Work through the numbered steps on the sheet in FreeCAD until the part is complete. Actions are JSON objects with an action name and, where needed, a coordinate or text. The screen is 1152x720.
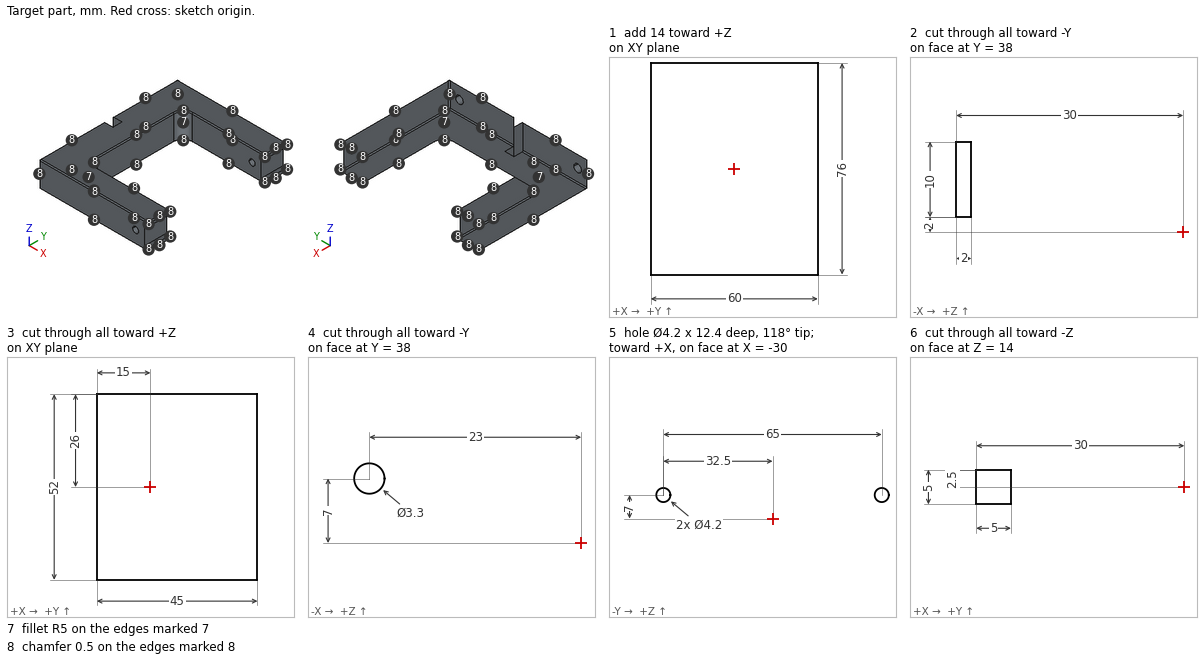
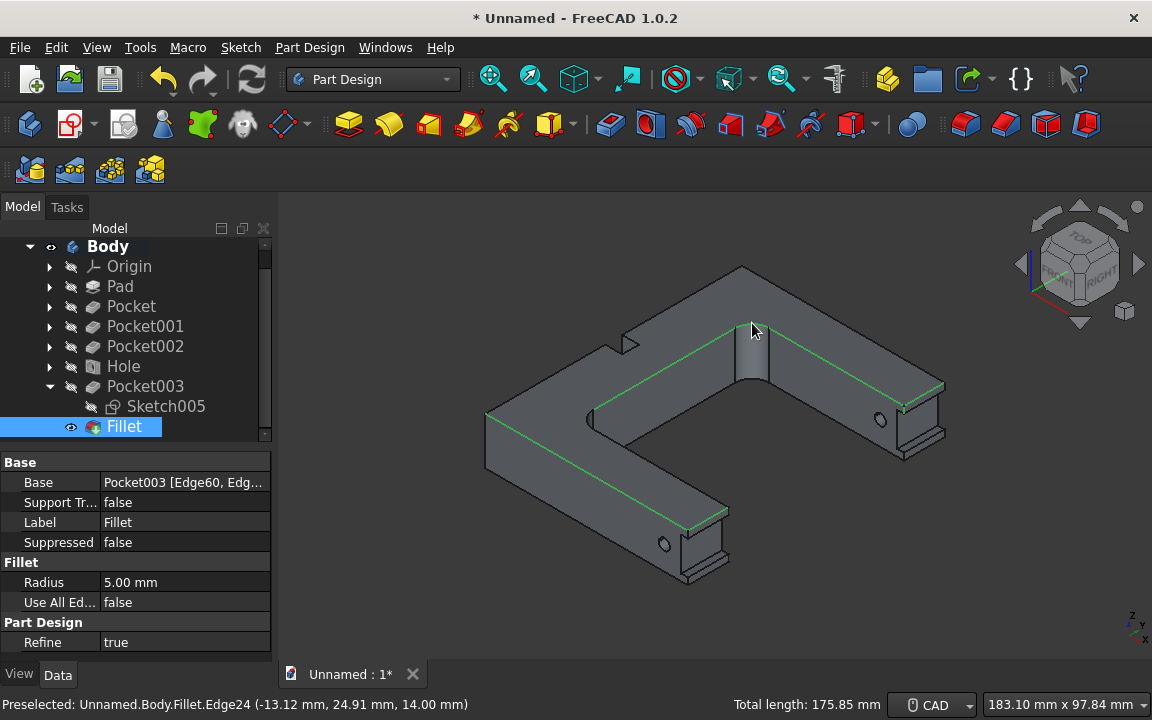
{"action": "left_click", "coordinate": [587, 419], "text": "ctrl"}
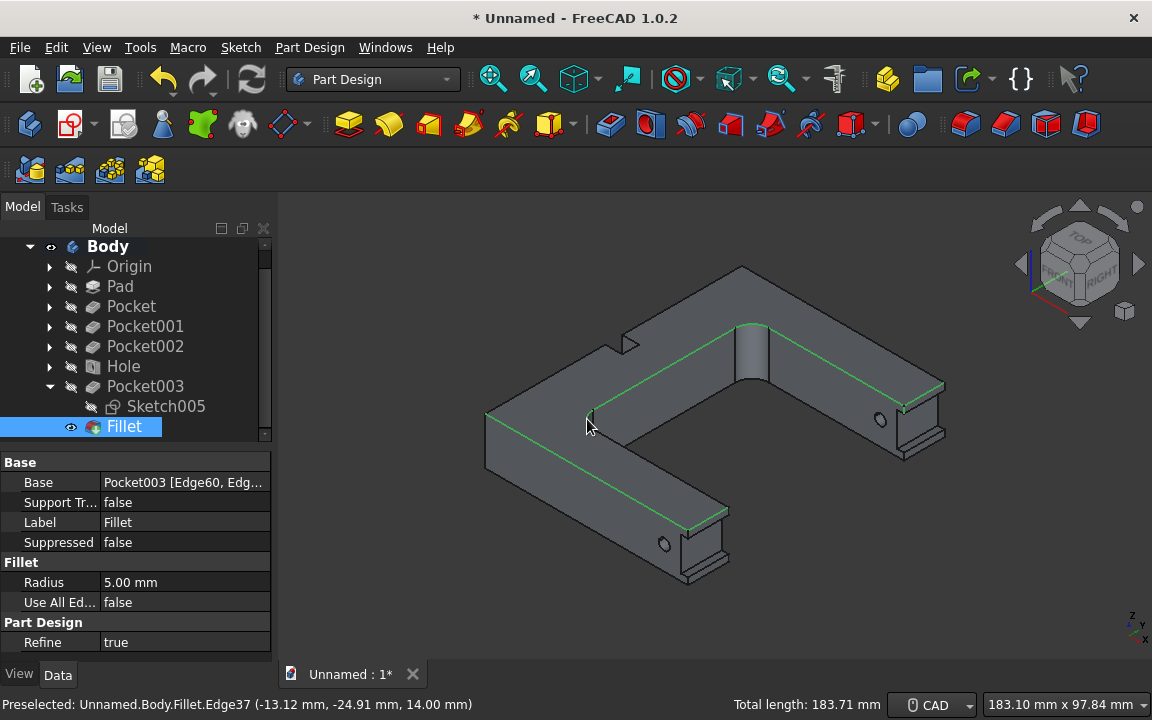
{"action": "key", "text": "2"}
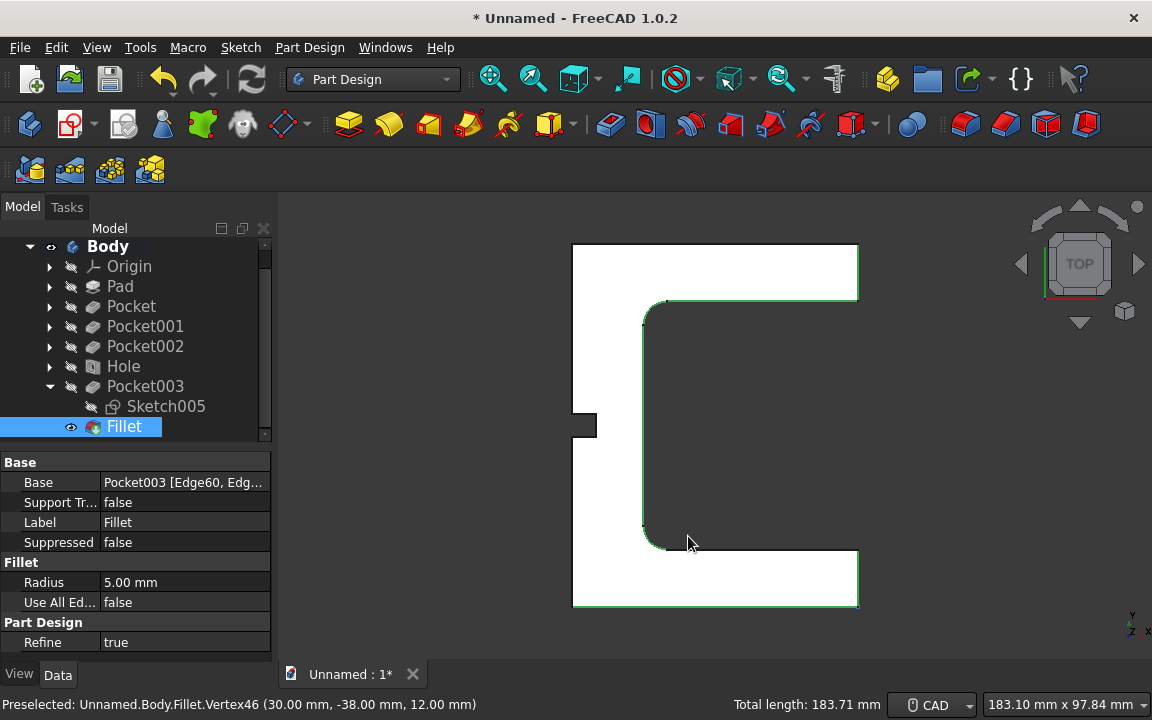
{"action": "left_click", "coordinate": [572, 328], "text": "ctrl"}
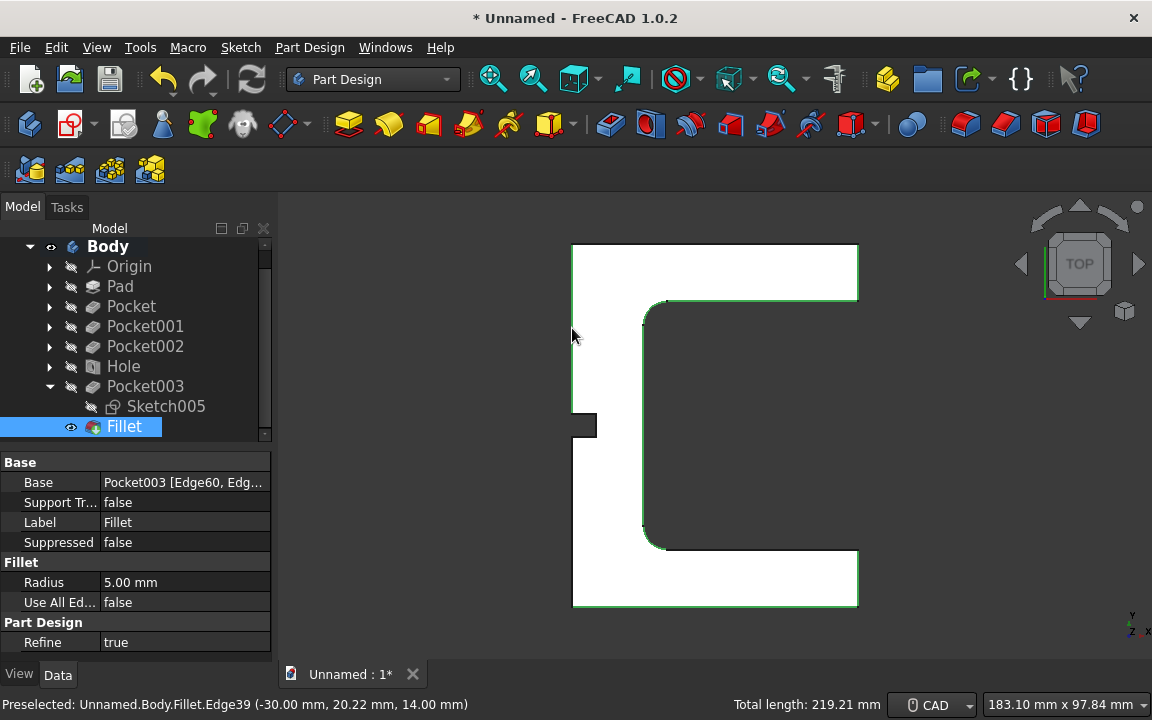
{"action": "left_click", "coordinate": [763, 549], "text": "ctrl"}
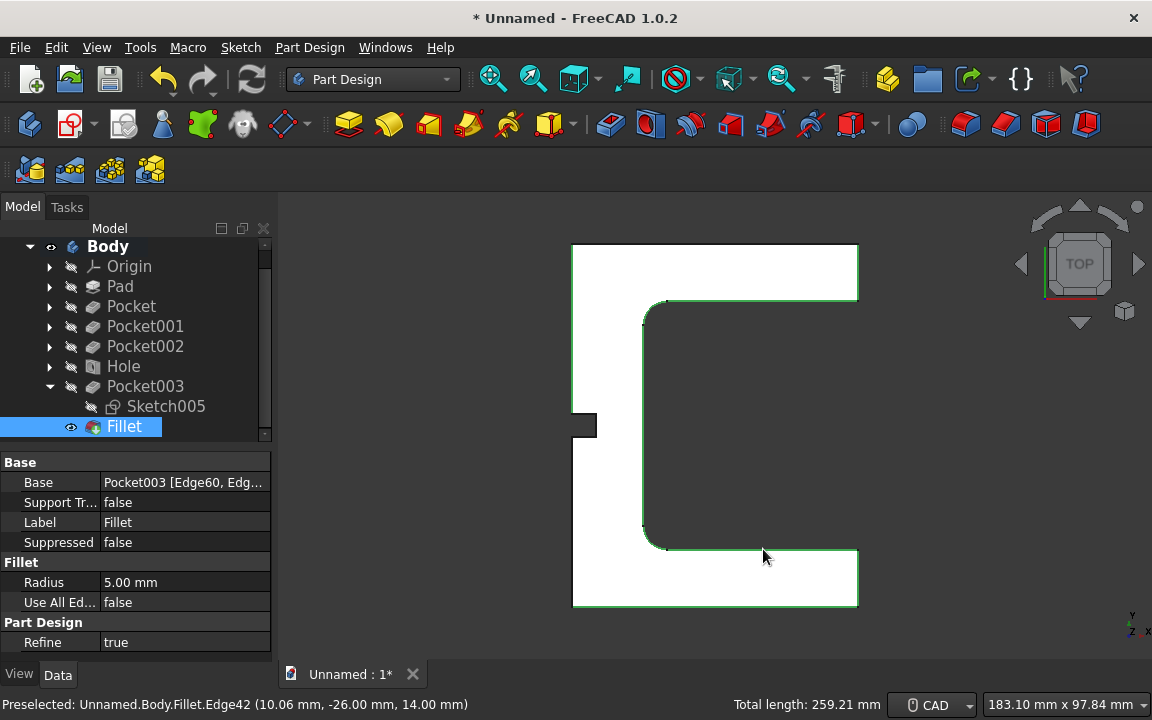
{"action": "left_click", "coordinate": [572, 521], "text": "ctrl"}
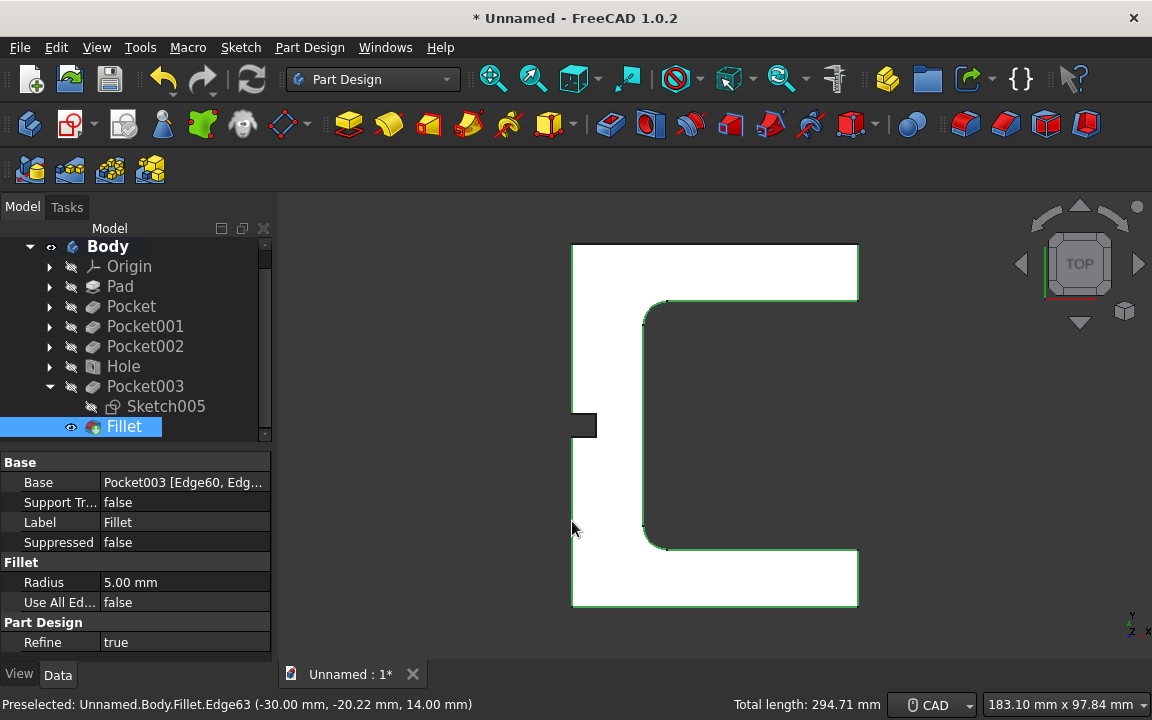
{"action": "left_click", "coordinate": [715, 243], "text": "ctrl"}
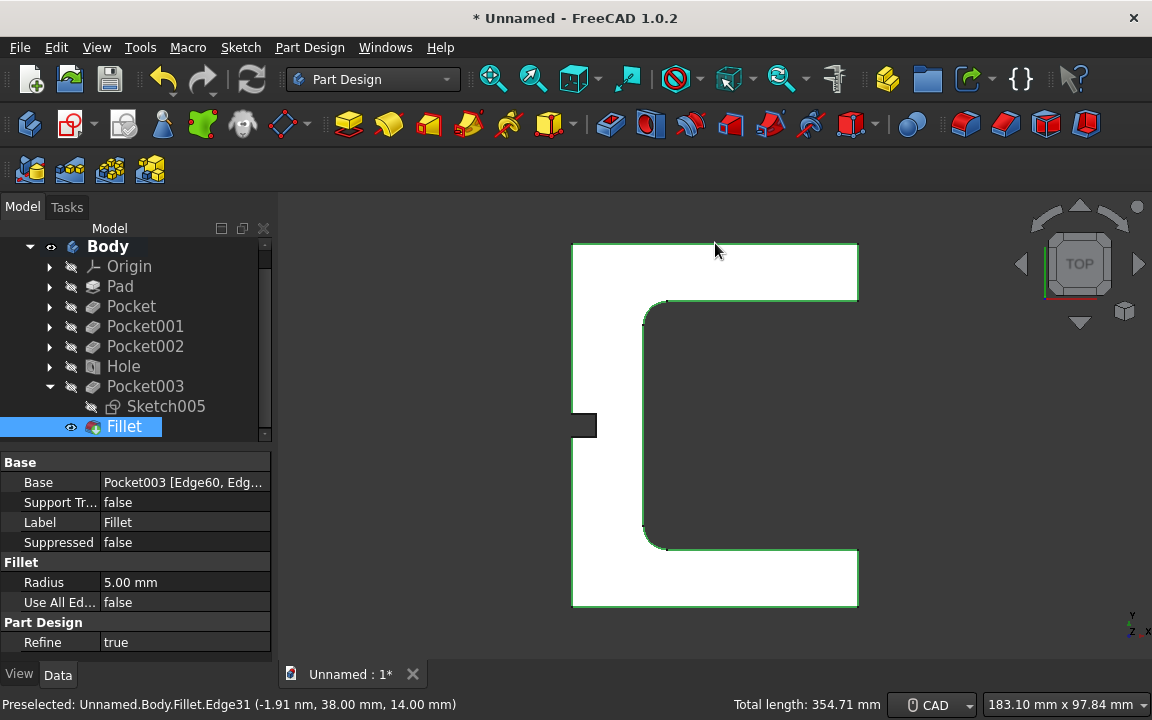
{"action": "scroll", "coordinate": [858, 606], "scroll_direction": "up", "scroll_amount": 8}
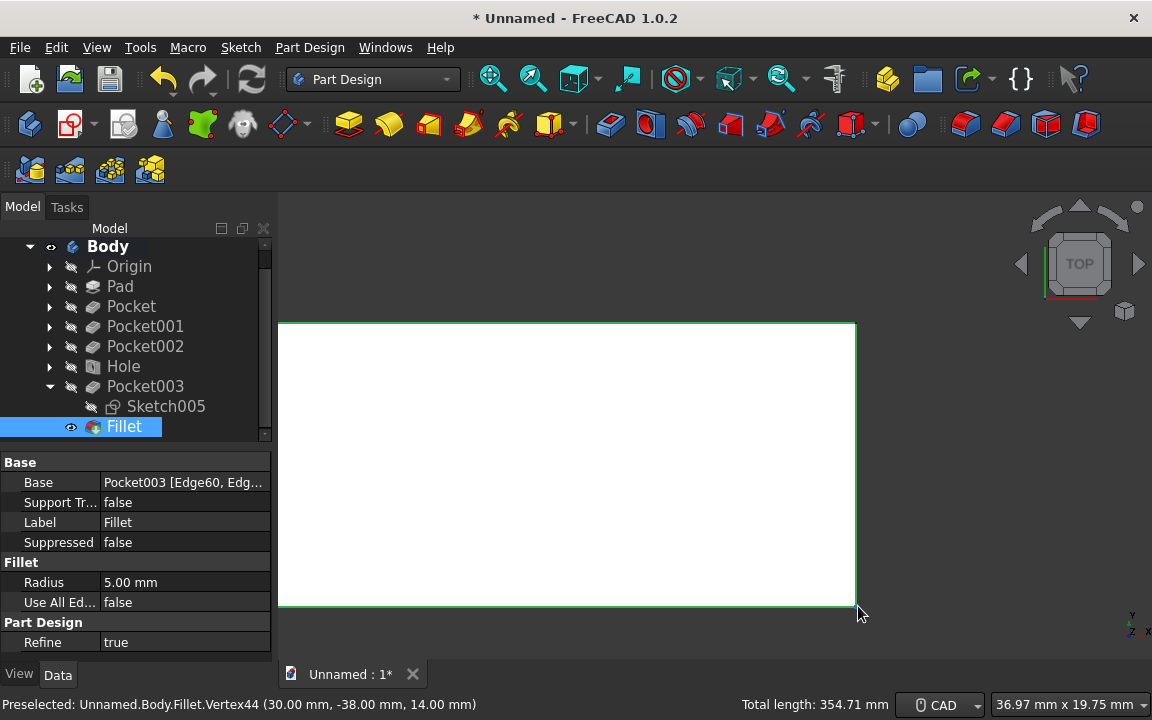
{"action": "left_click", "coordinate": [494, 80]}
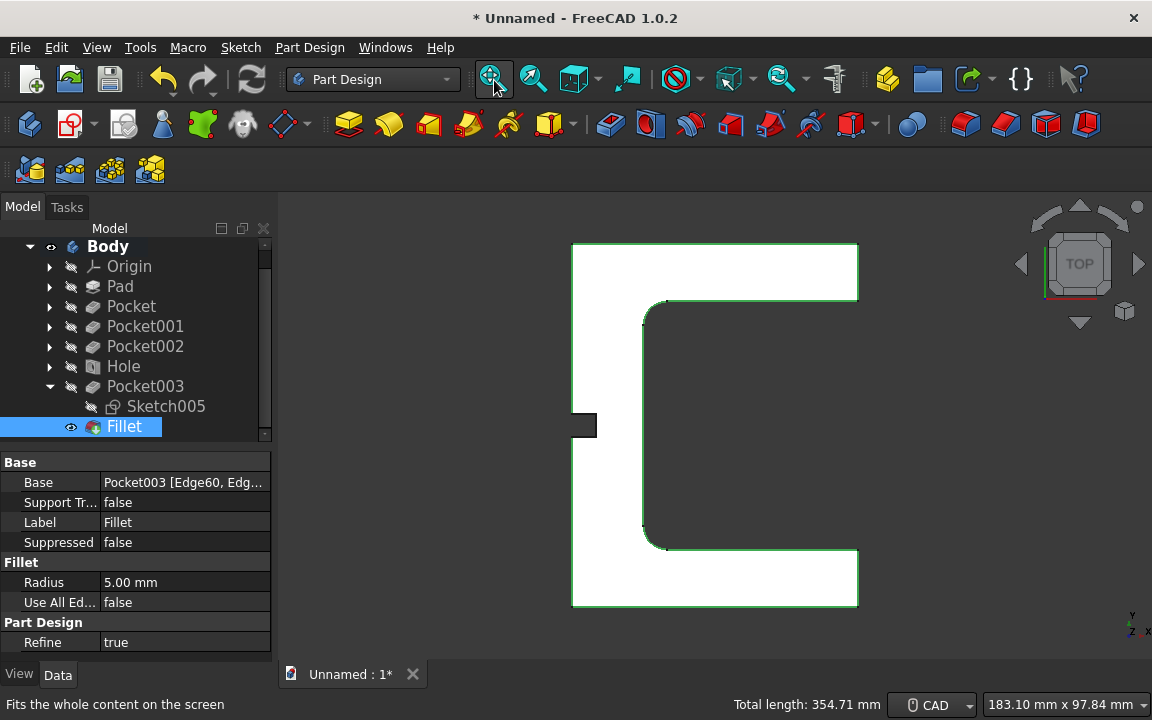
{"action": "key", "text": "0"}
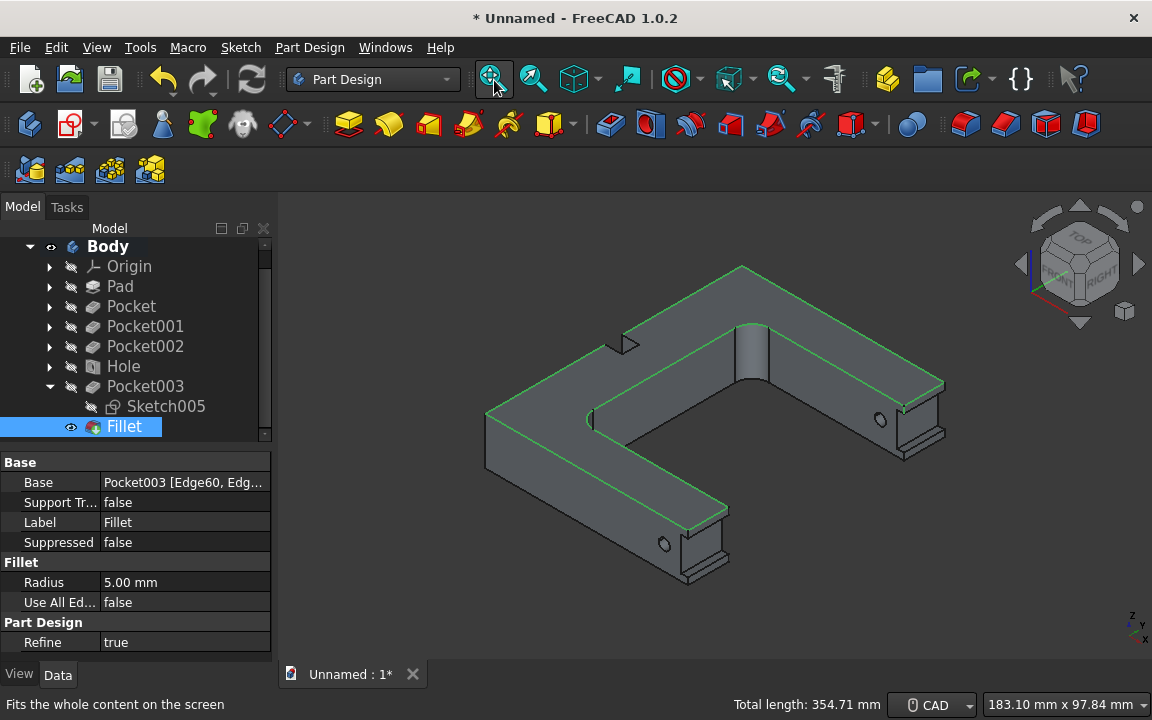
{"action": "scroll", "coordinate": [688, 580], "scroll_direction": "up", "scroll_amount": 8}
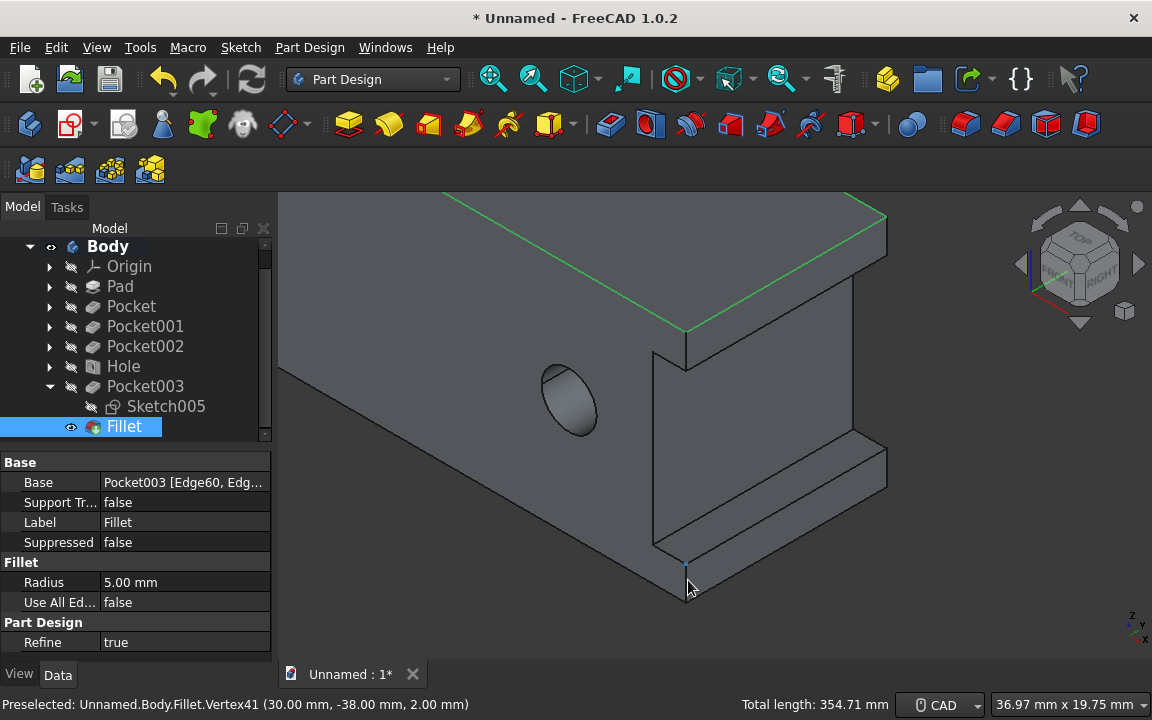
{"action": "left_click", "coordinate": [686, 583], "text": "ctrl"}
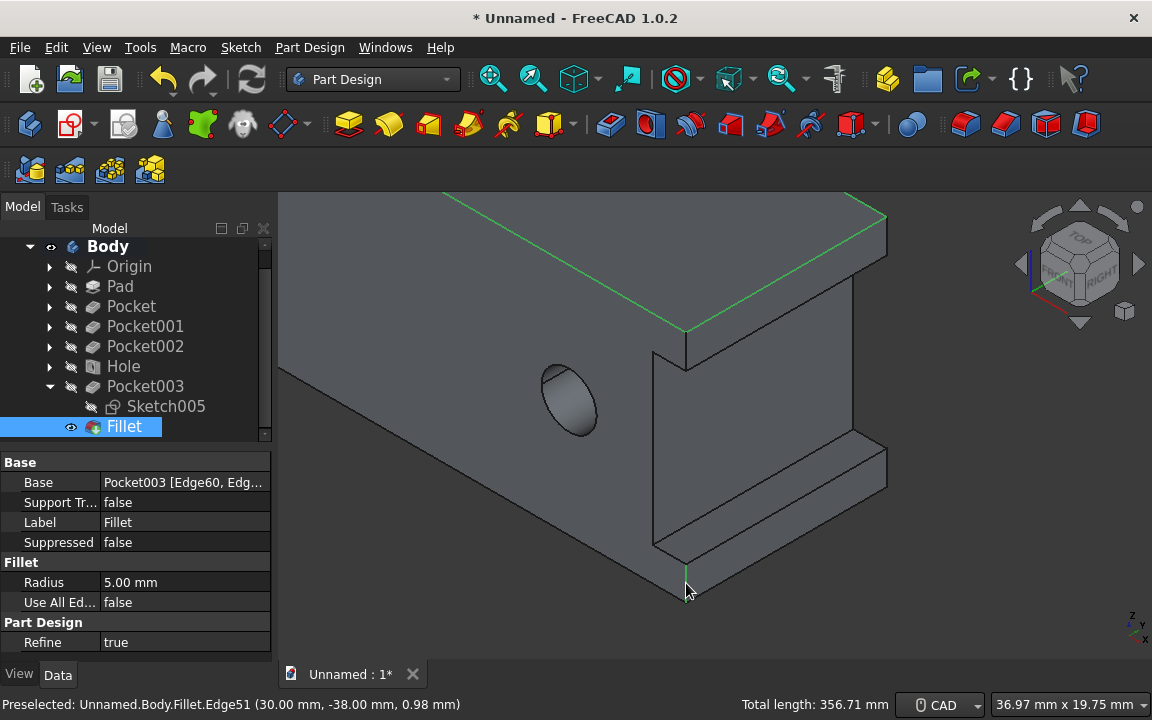
{"action": "left_click", "coordinate": [686, 351], "text": "ctrl"}